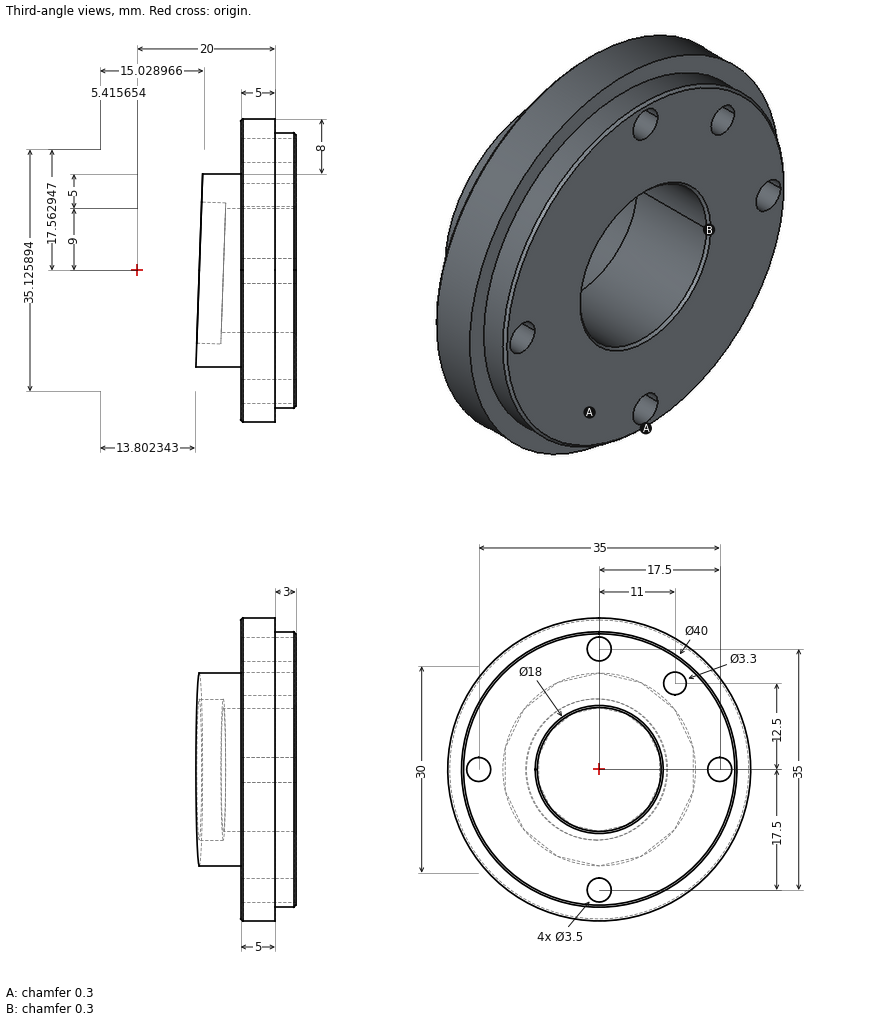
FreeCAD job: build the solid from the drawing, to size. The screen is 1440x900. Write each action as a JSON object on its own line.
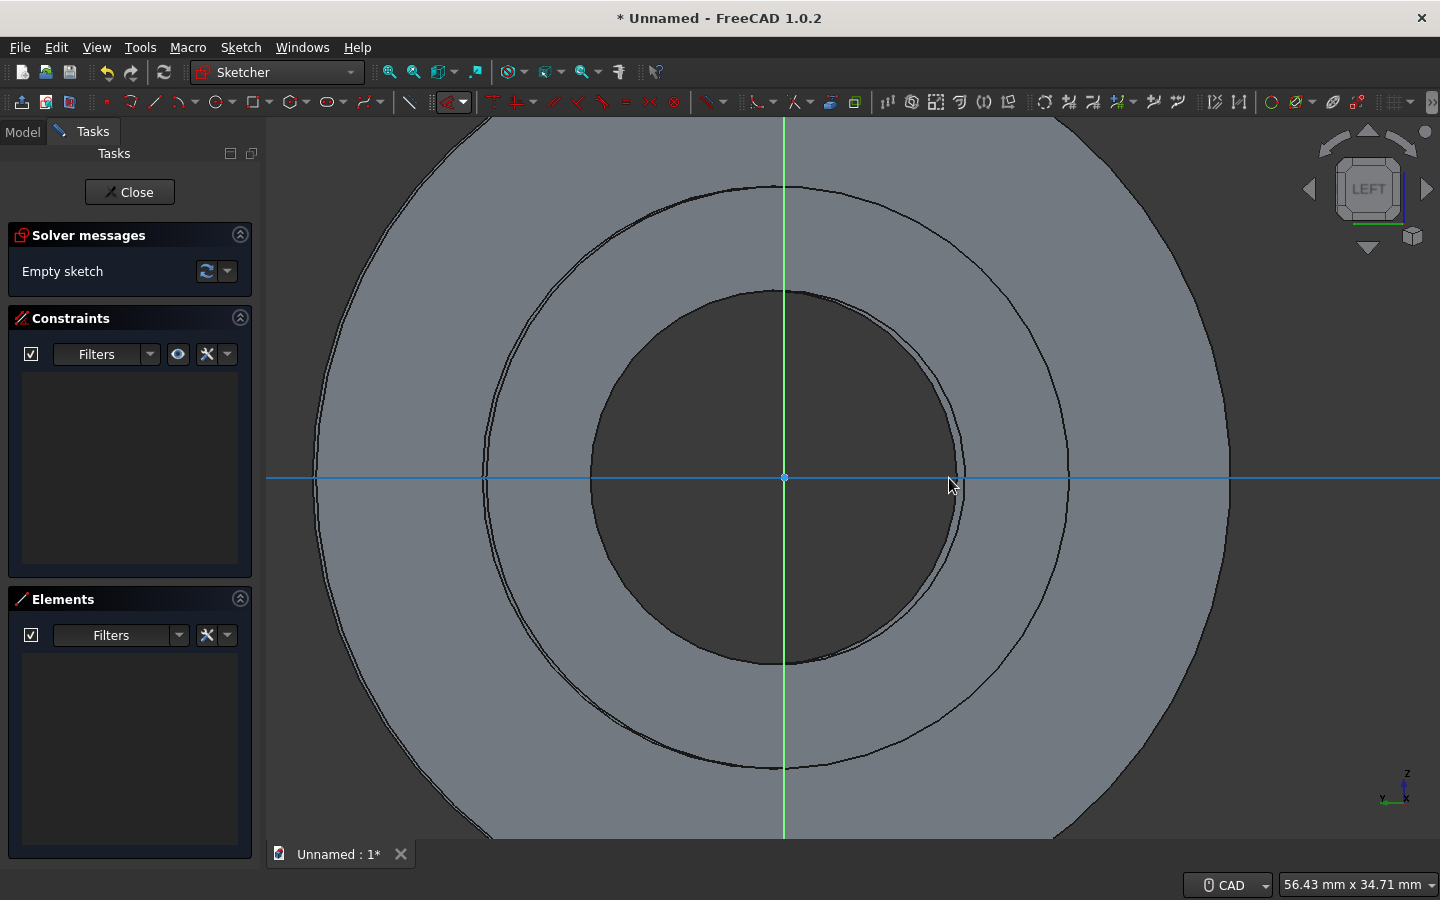
{"action": "left_click", "coordinate": [216, 102]}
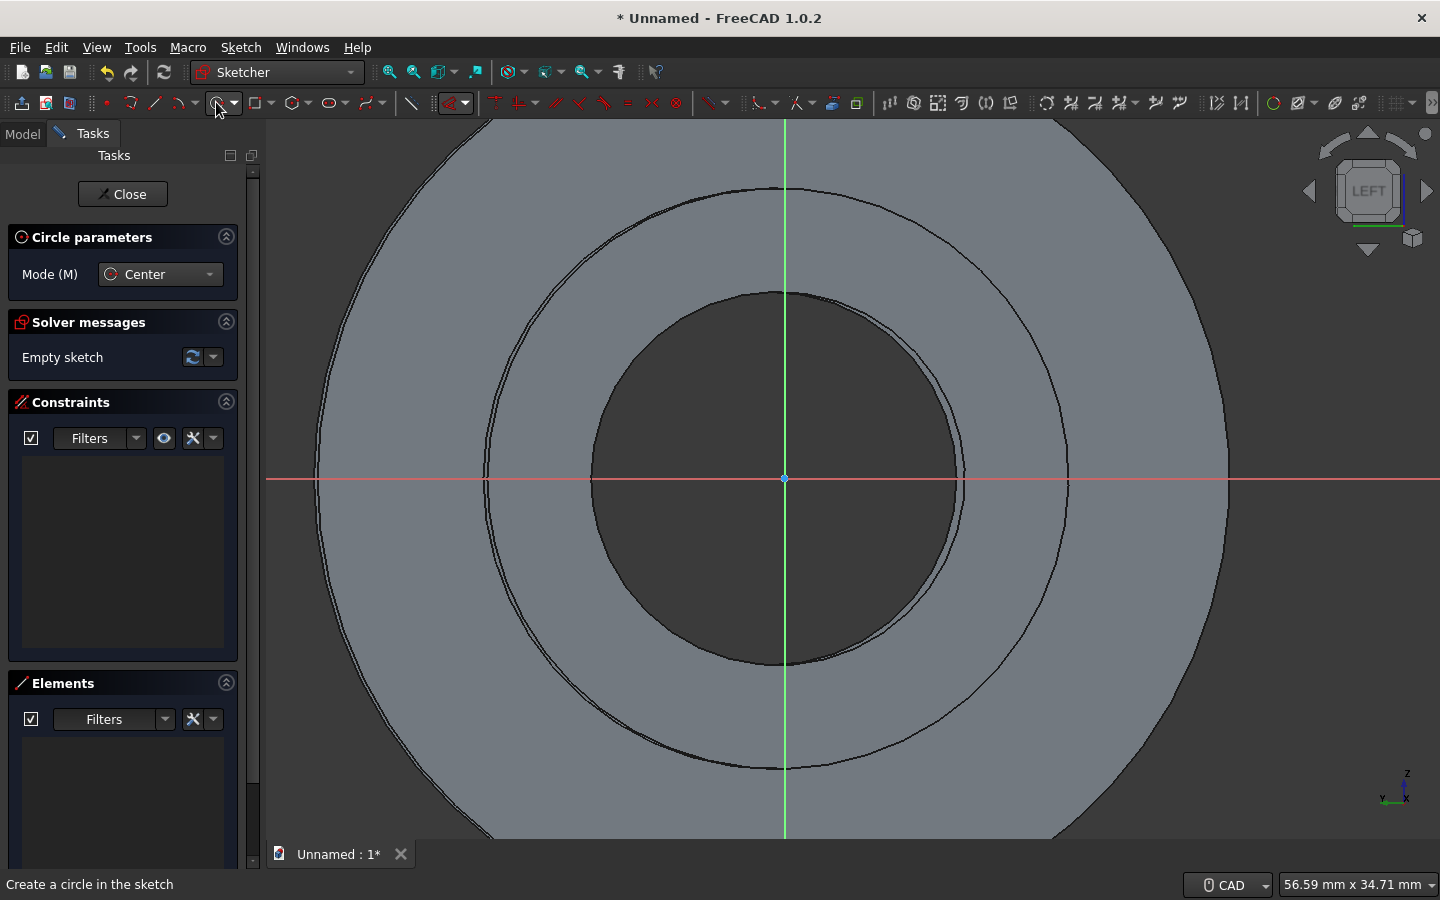
{"action": "left_click", "coordinate": [785, 479]}
{"action": "mouse_move", "coordinate": [935, 328]}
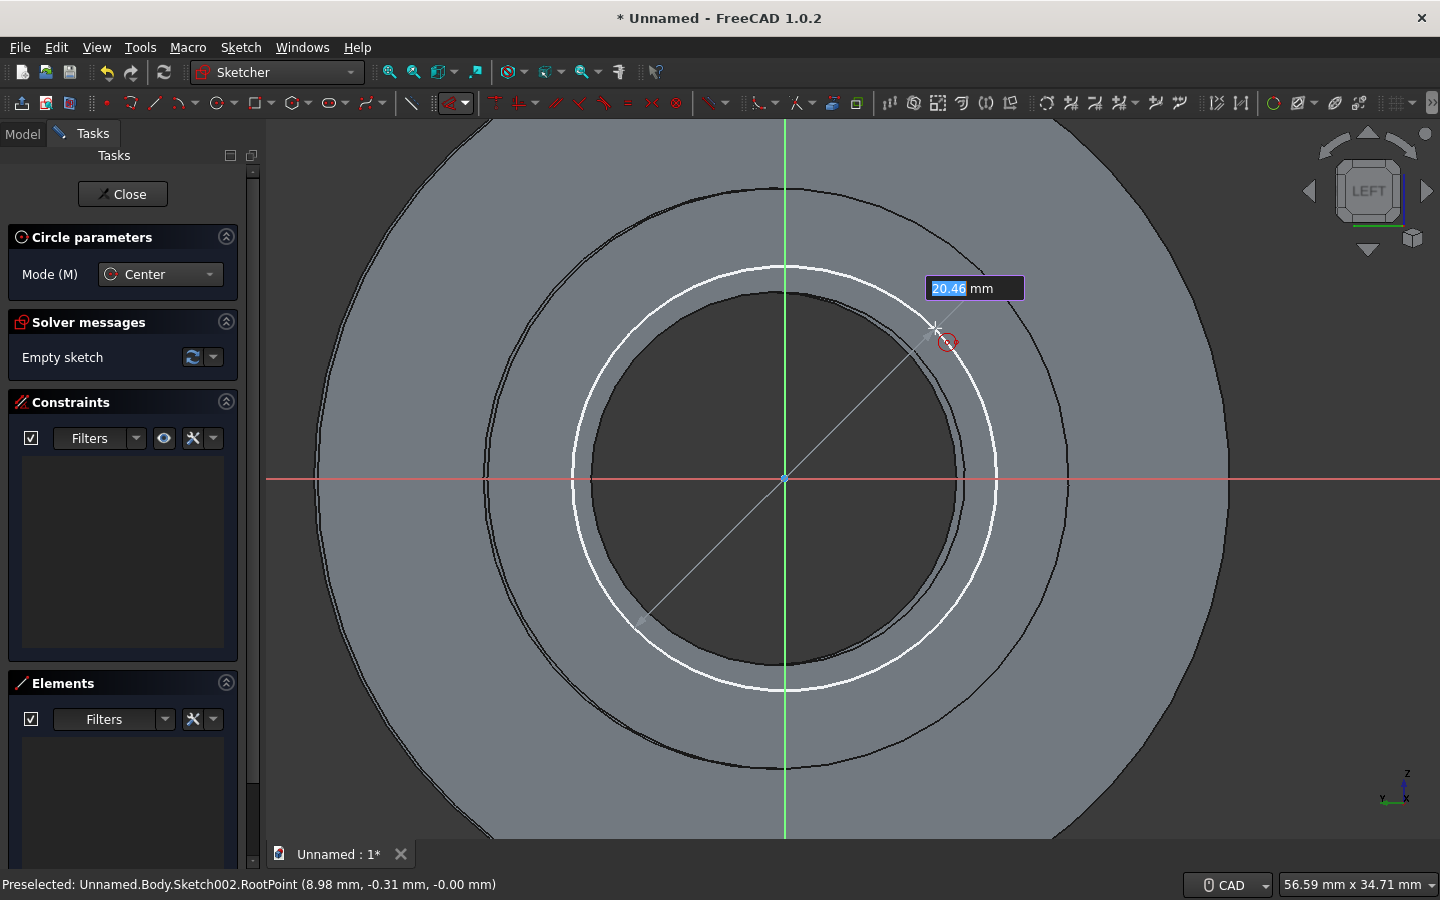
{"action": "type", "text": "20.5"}
{"action": "key", "text": "Return"}
{"action": "key", "text": "Escape"}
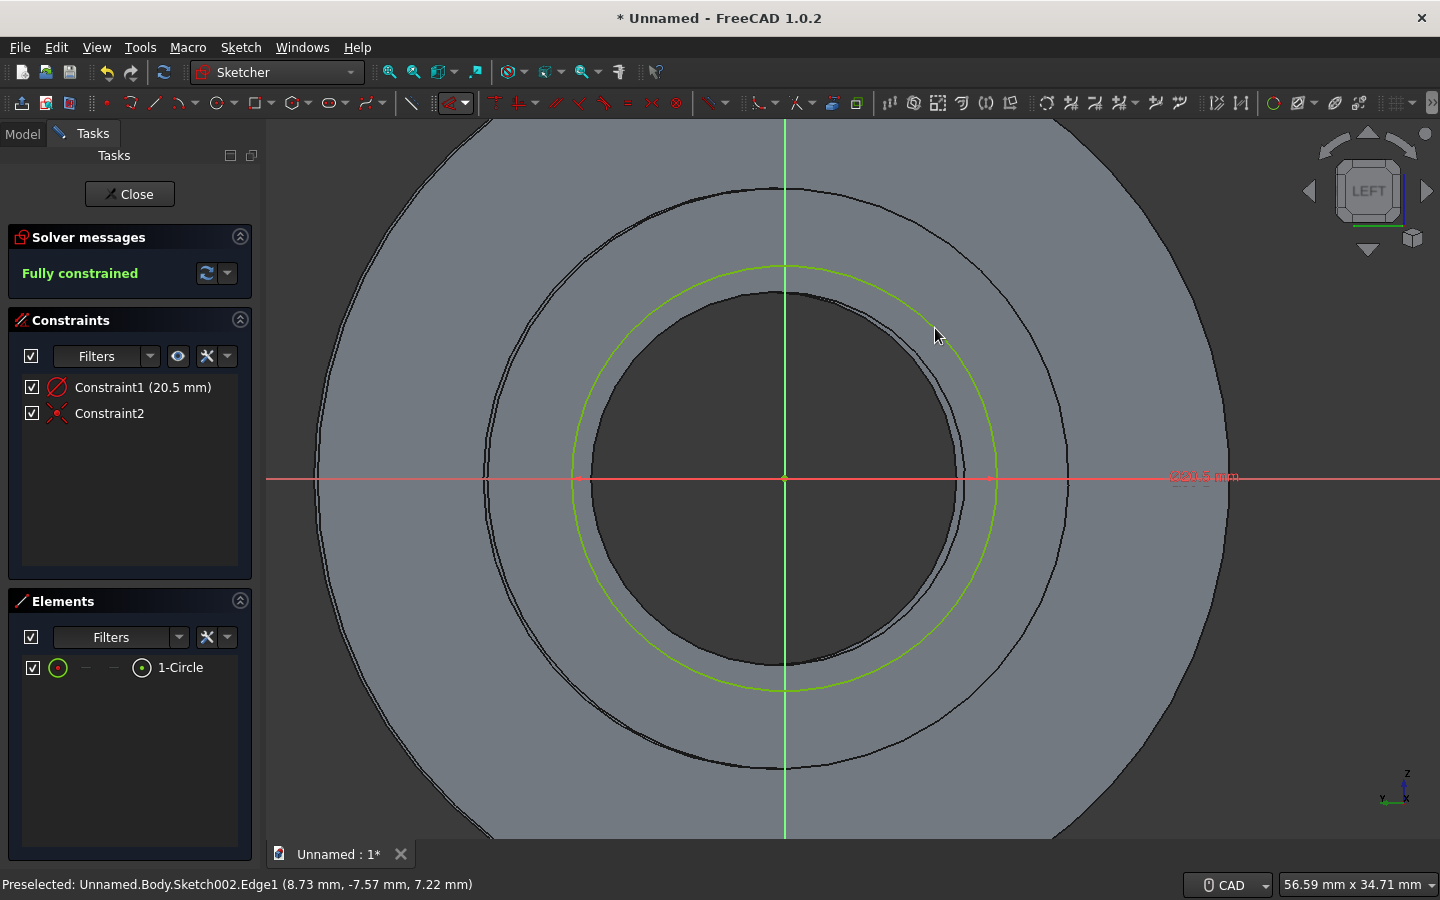
{"action": "left_click", "coordinate": [130, 194]}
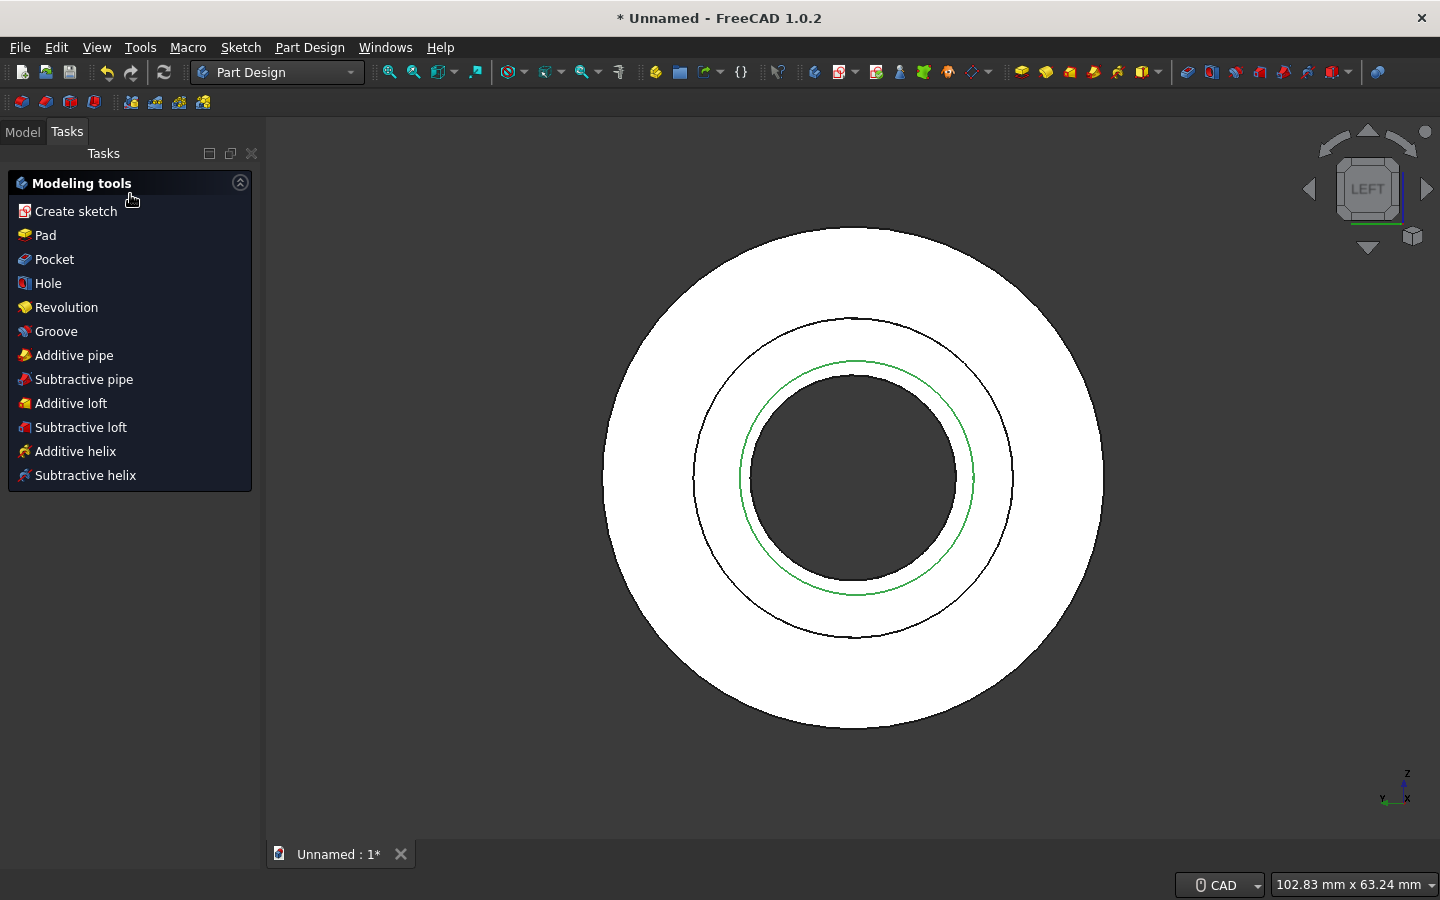
{"action": "left_click", "coordinate": [1188, 72]}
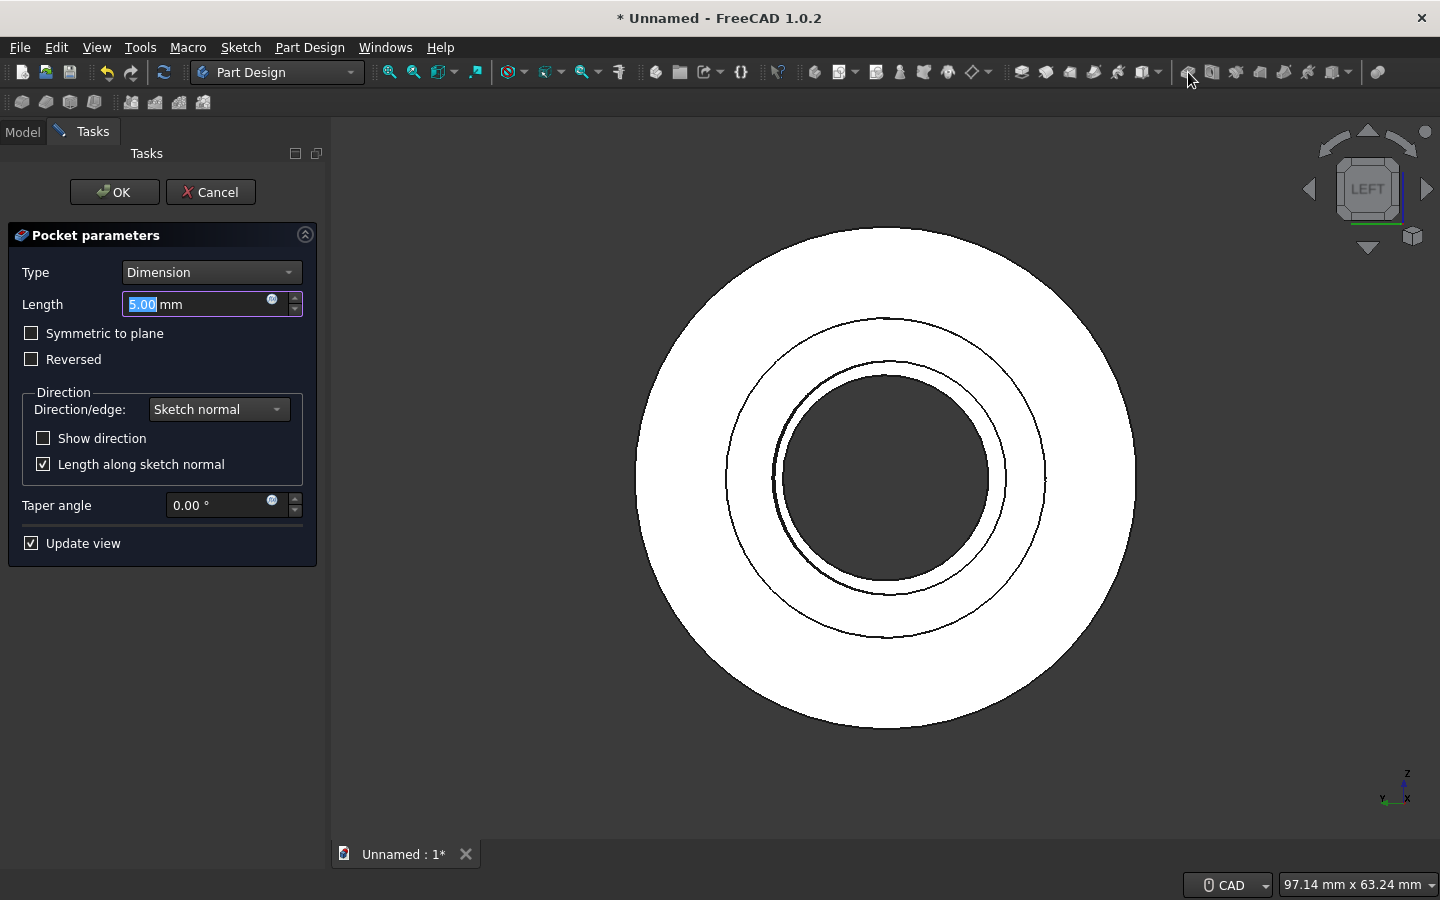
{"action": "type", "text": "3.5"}
{"action": "key", "text": "Tab"}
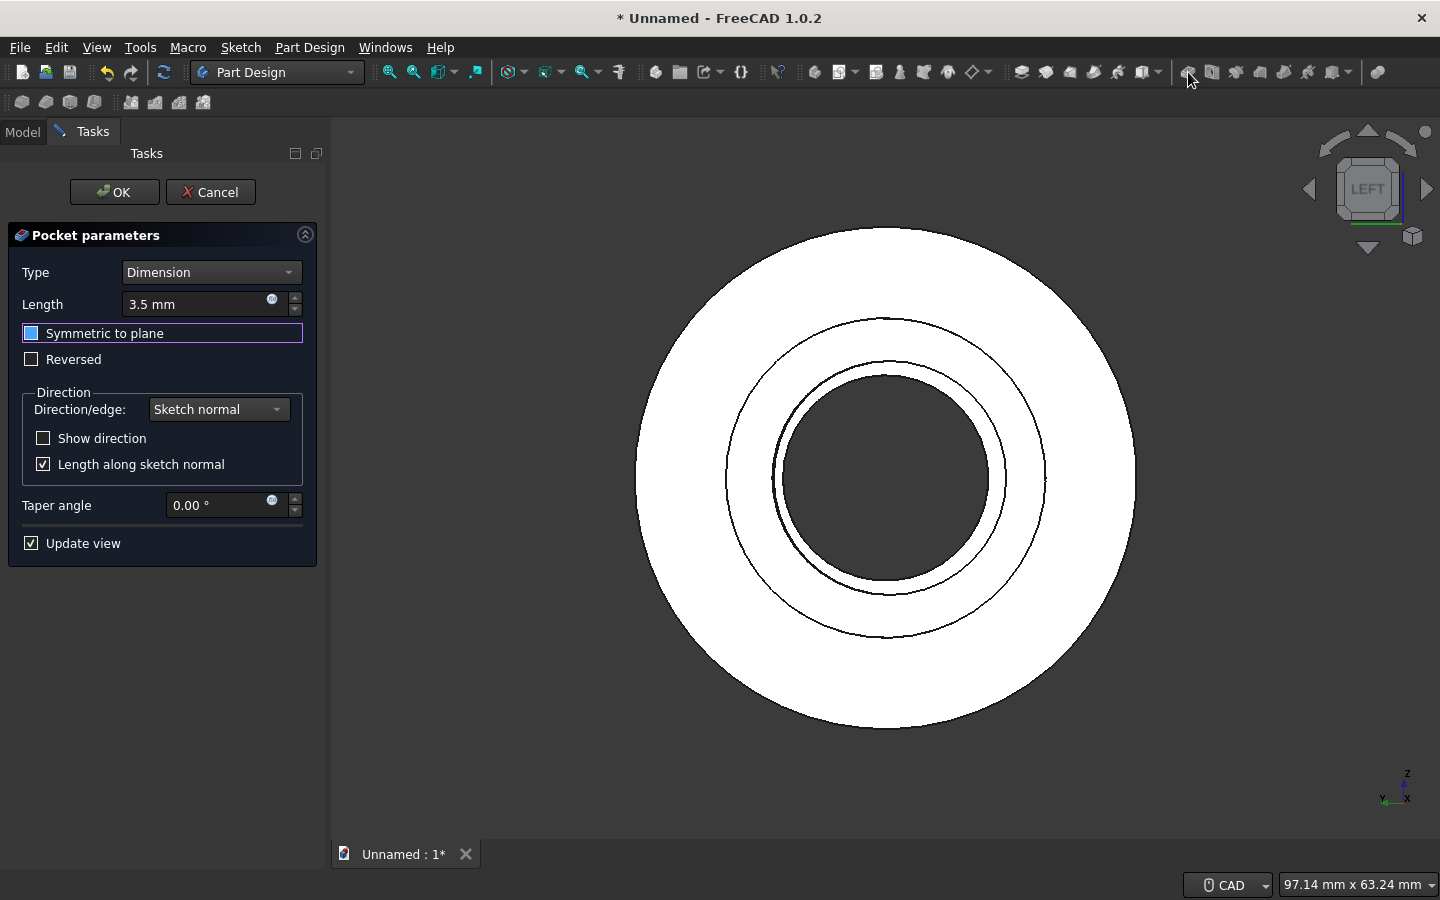
{"action": "left_click", "coordinate": [115, 192]}